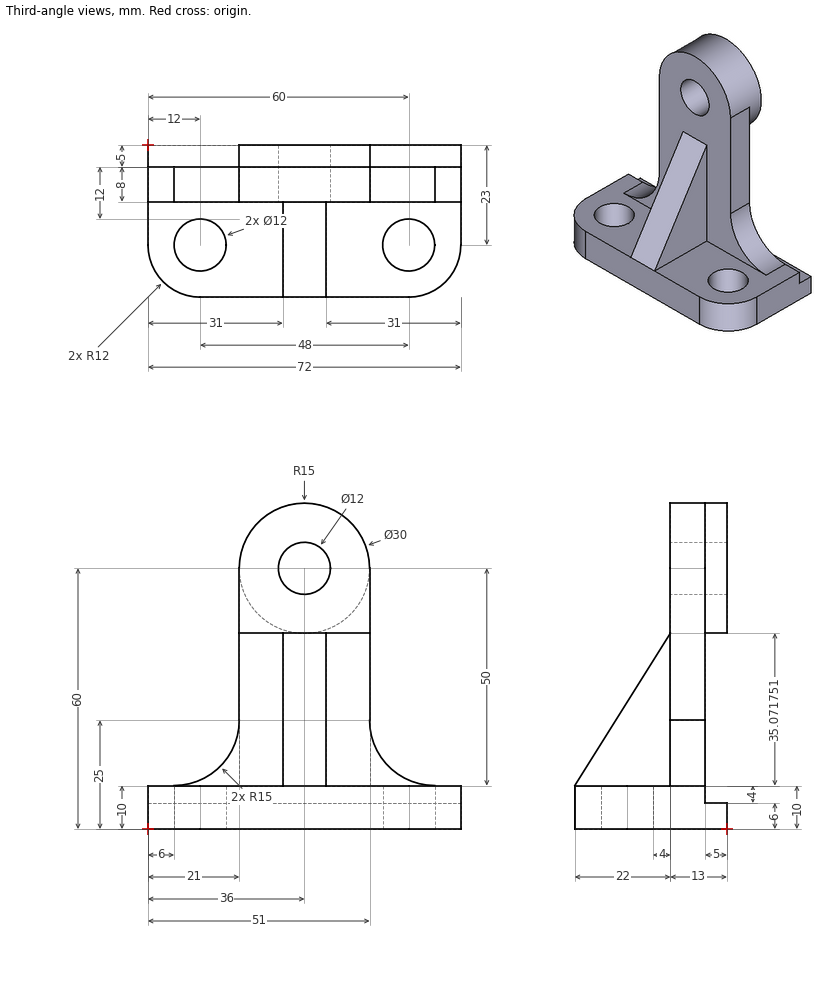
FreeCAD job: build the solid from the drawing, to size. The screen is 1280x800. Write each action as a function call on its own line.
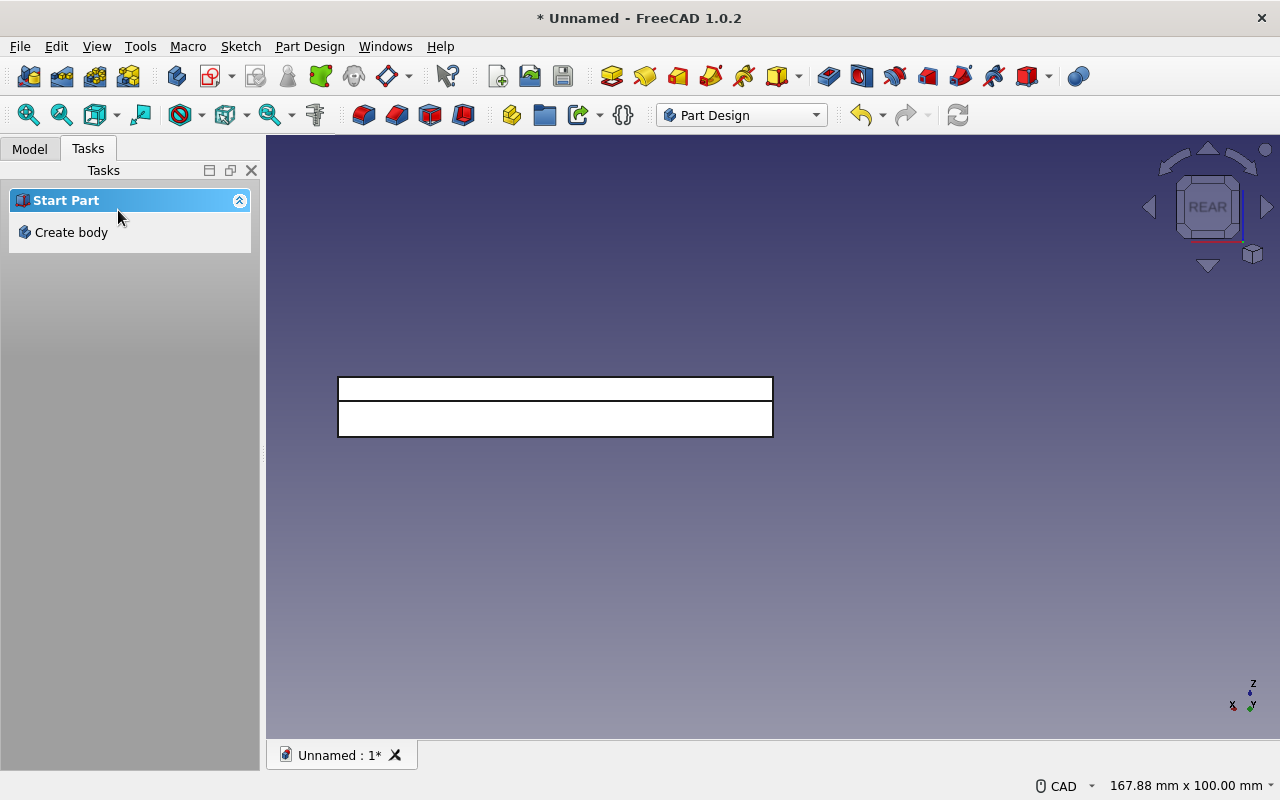
click(29, 116)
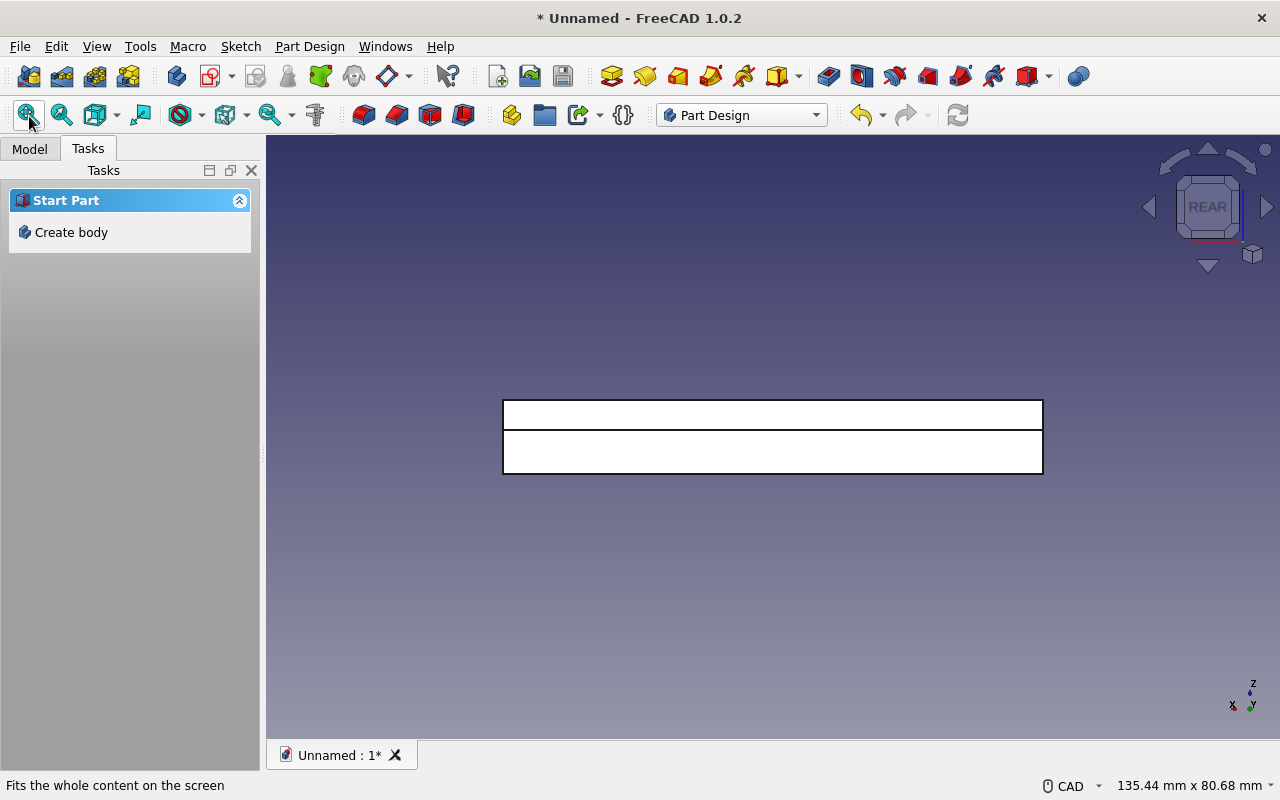
click(542, 414)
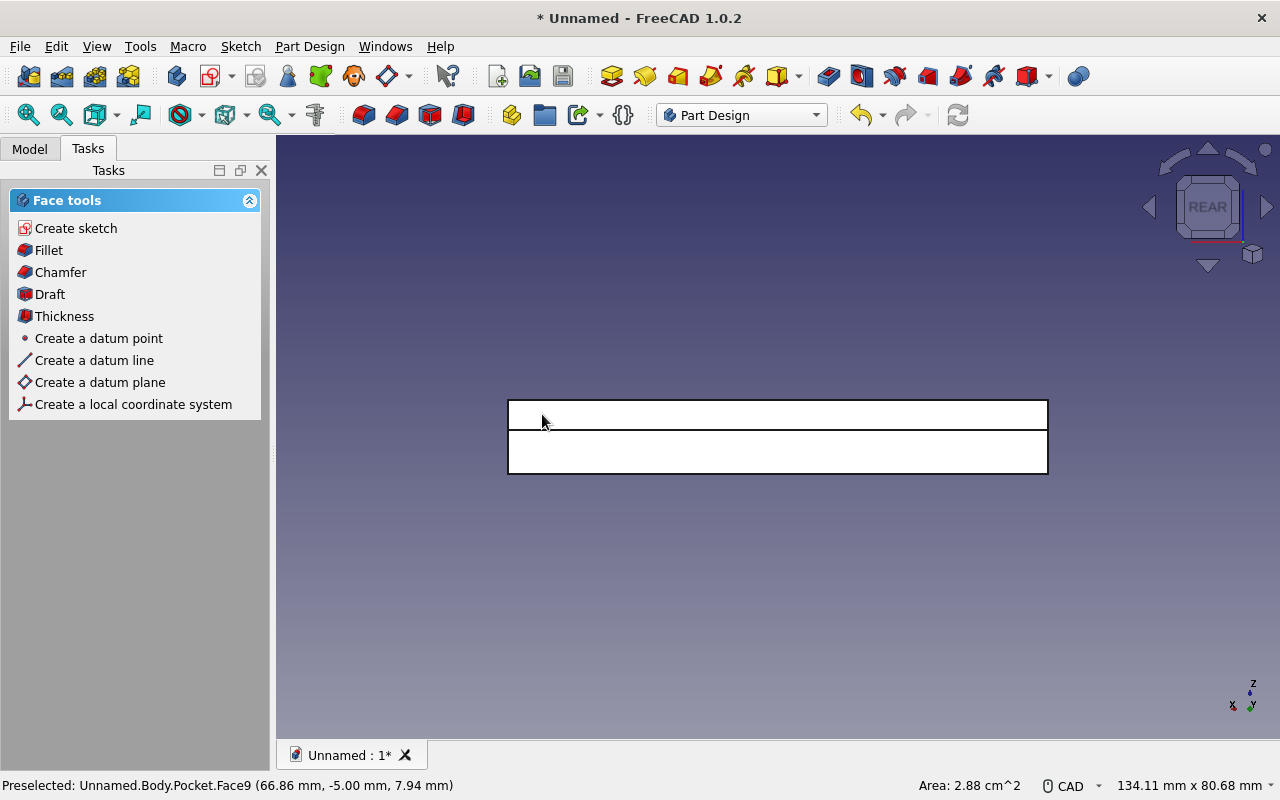
click(210, 76)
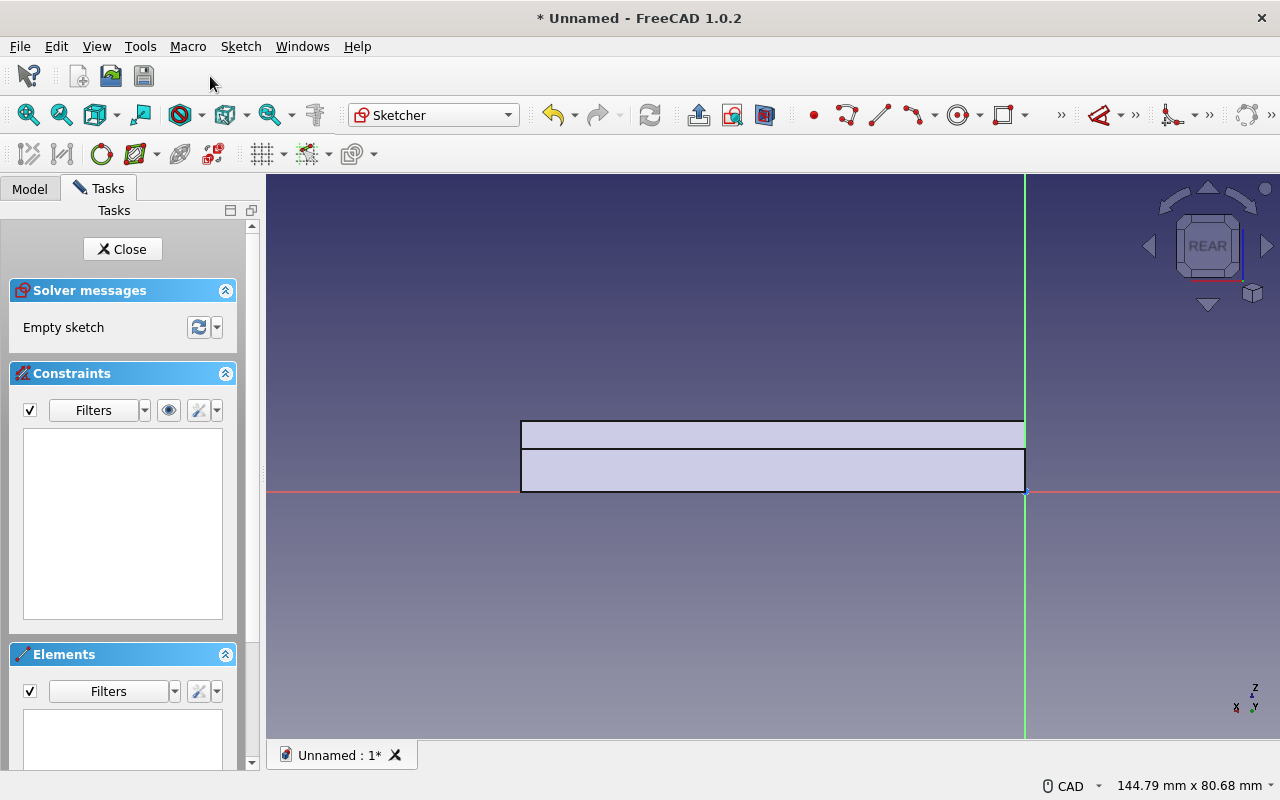
scroll(532, 711, down, 3)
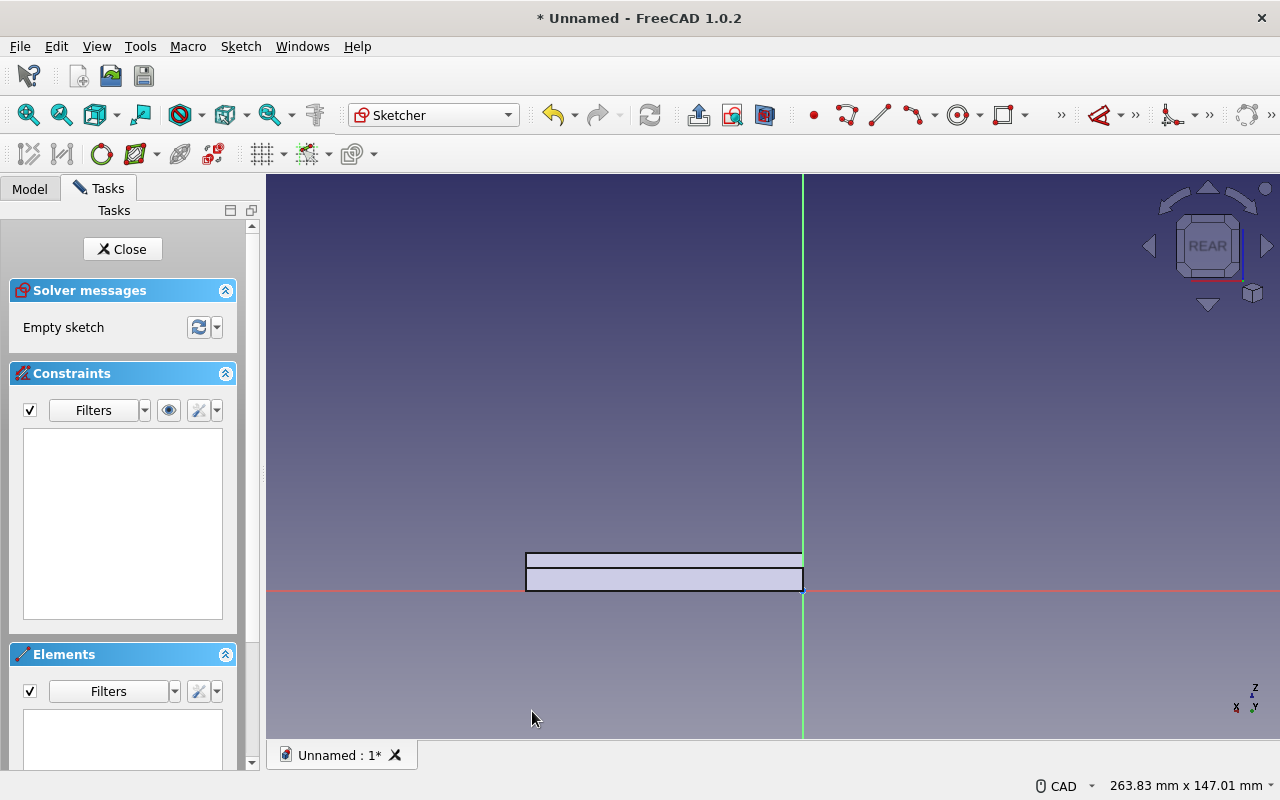
click(847, 116)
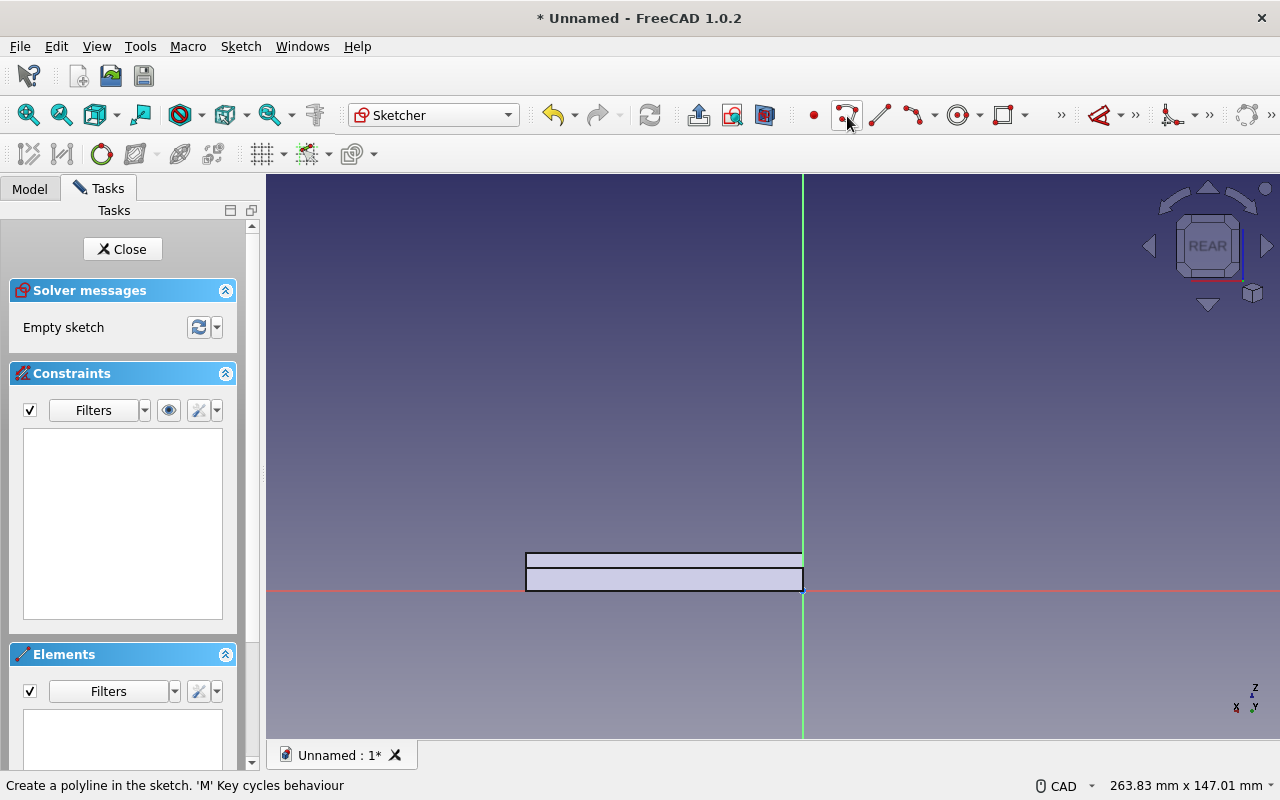
click(607, 360)
click(607, 553)
click(722, 553)
click(722, 360)
right_click(722, 360)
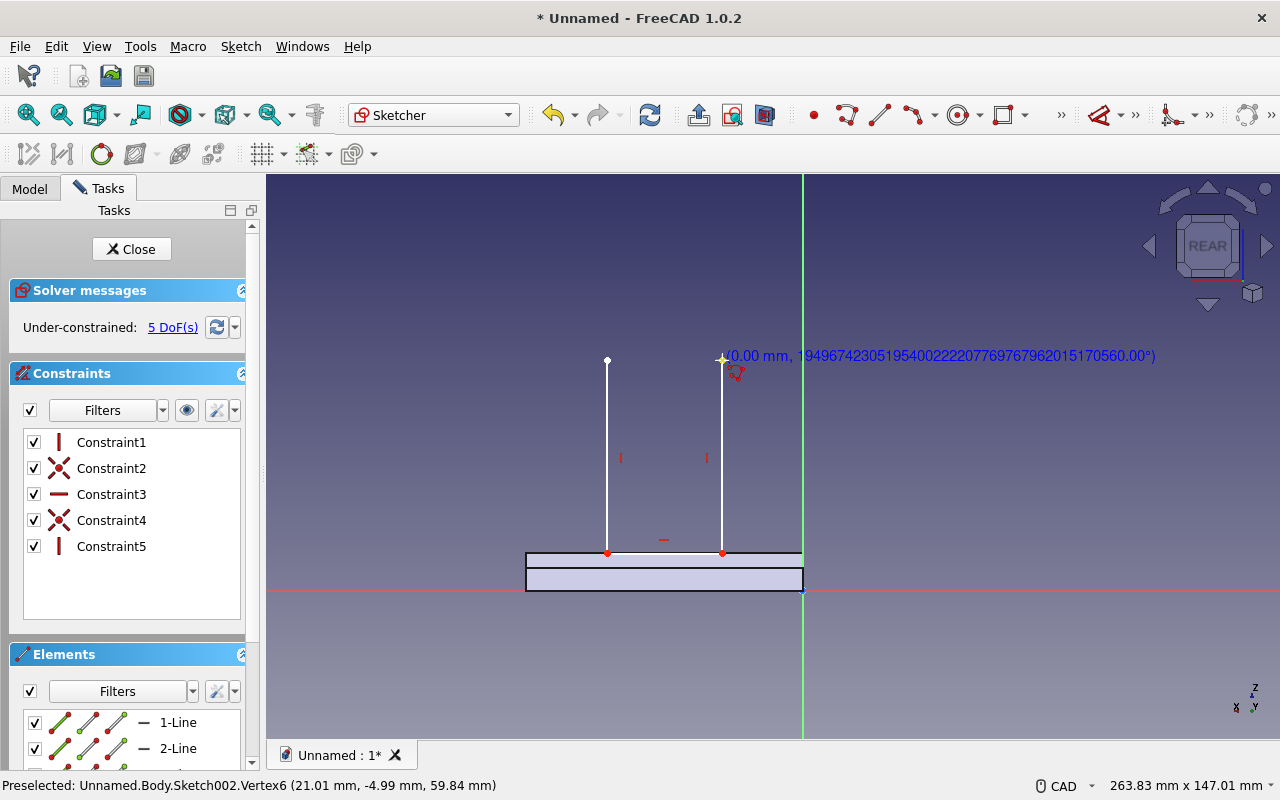
click(912, 116)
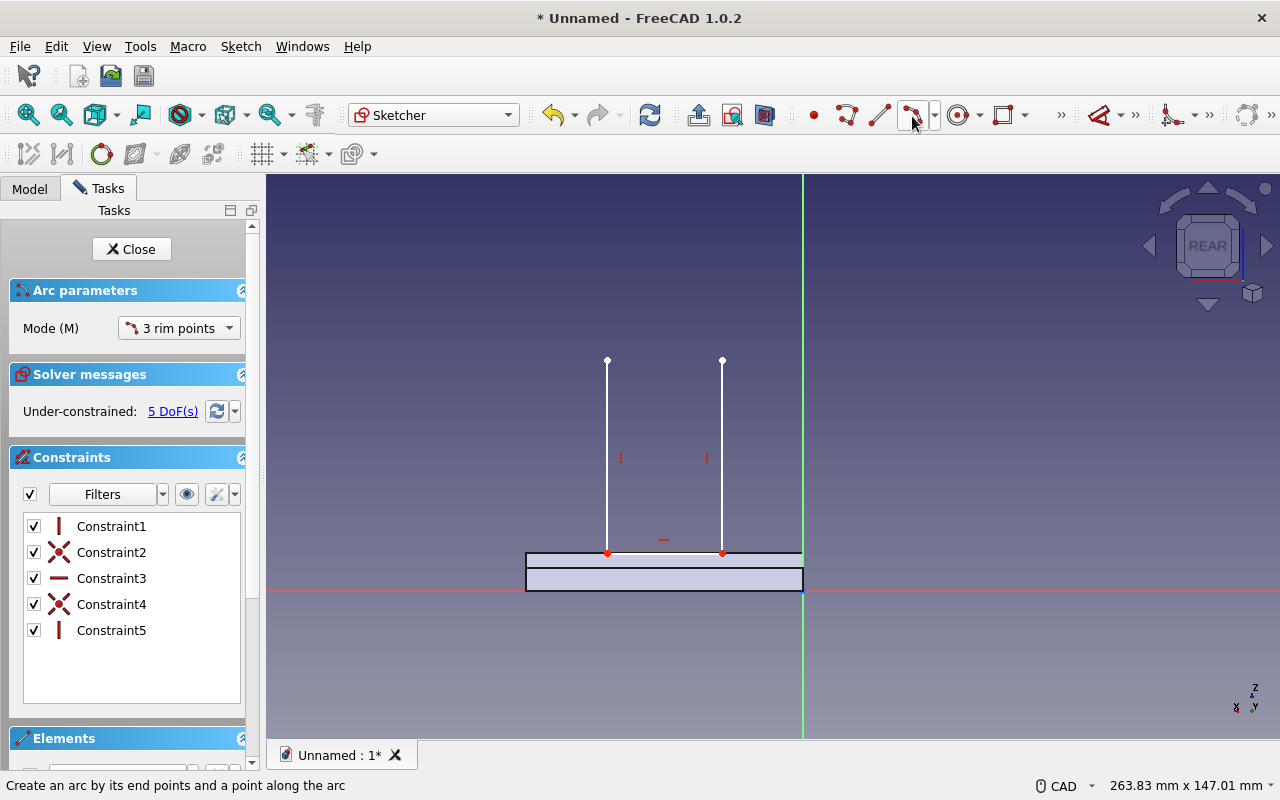
click(722, 361)
click(607, 361)
click(664, 303)
key(Escape)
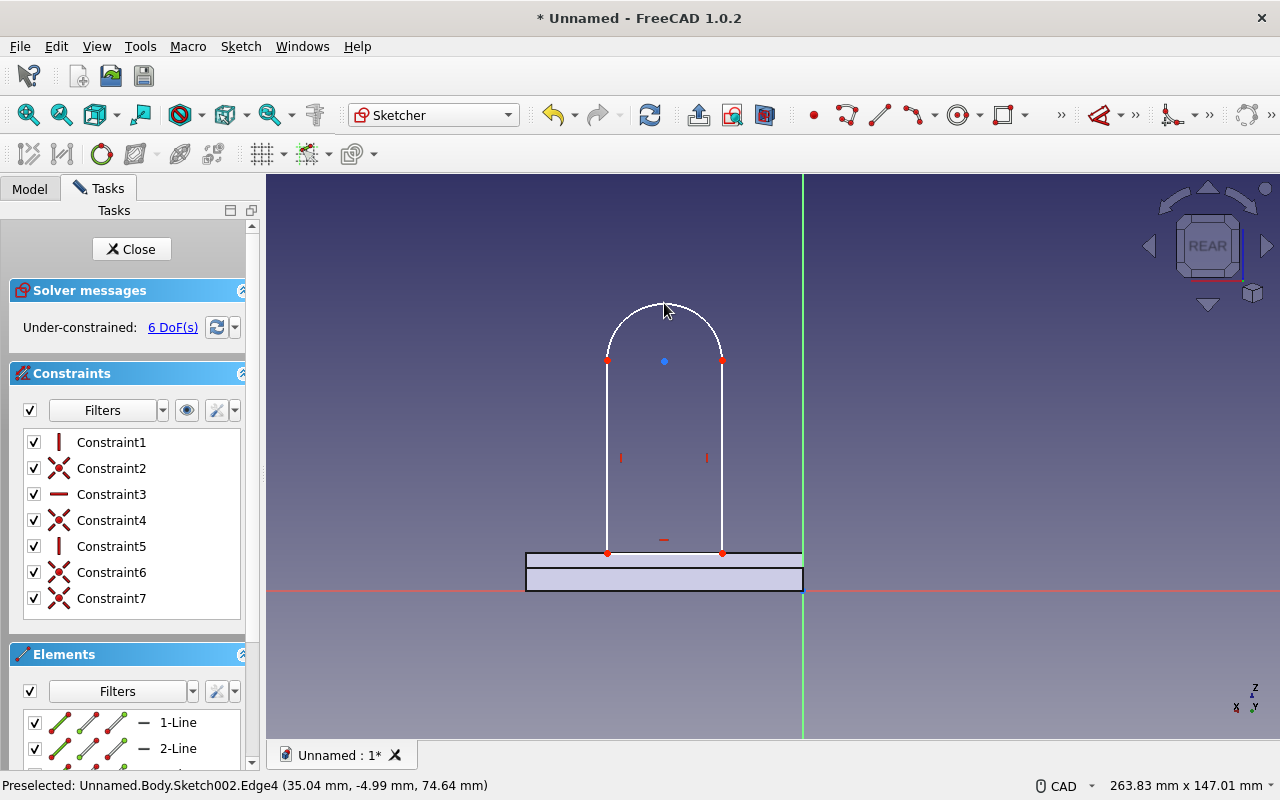
click(607, 419)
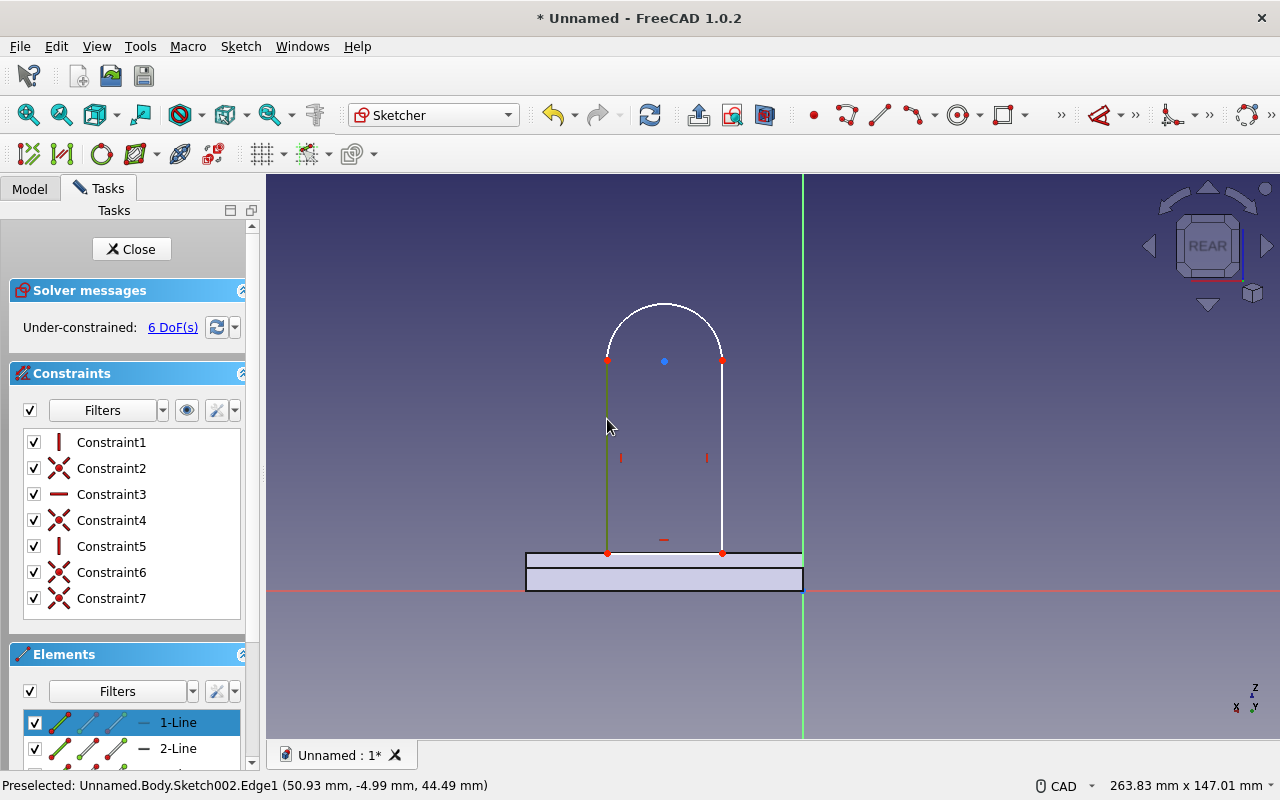
click(698, 315)